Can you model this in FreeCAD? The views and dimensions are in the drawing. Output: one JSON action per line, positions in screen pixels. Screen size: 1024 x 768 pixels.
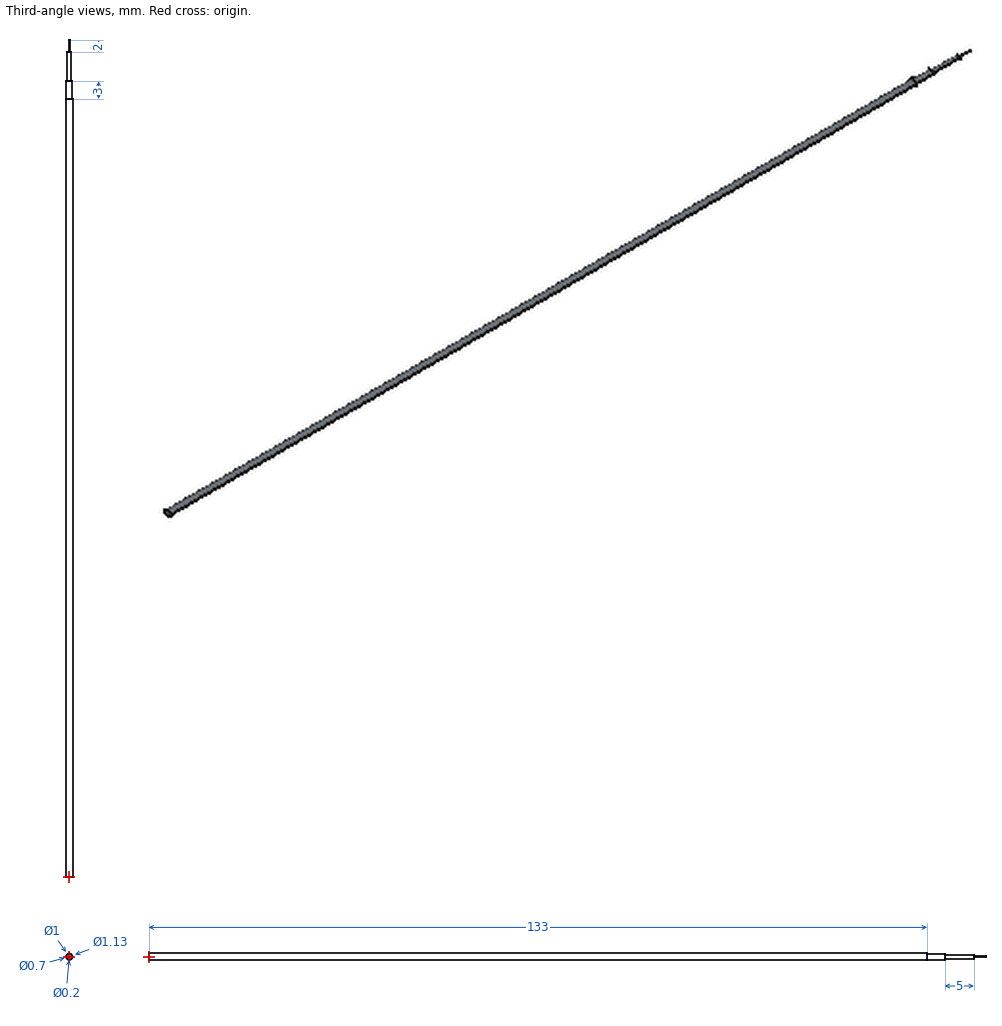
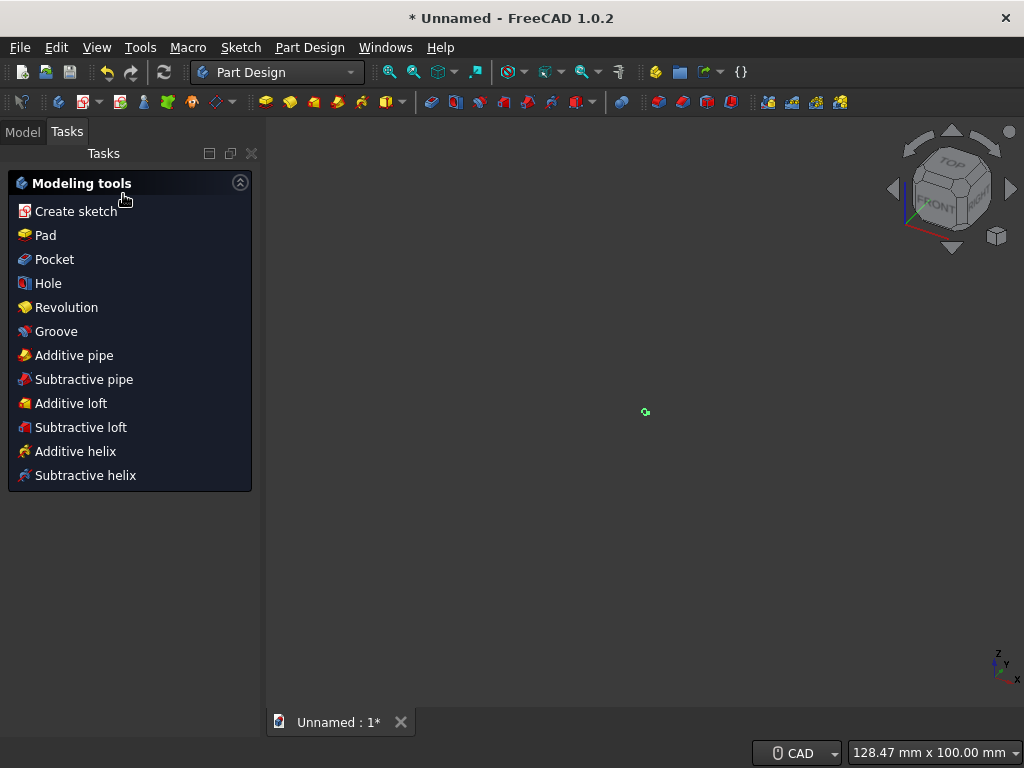
{"action": "left_click", "coordinate": [266, 102]}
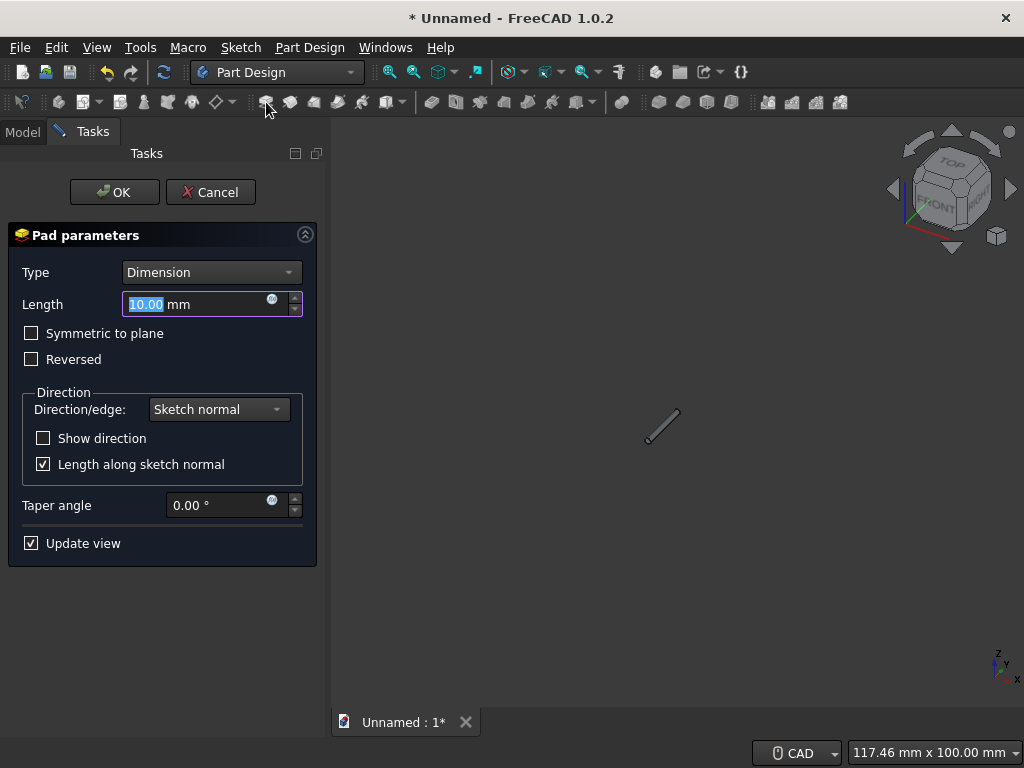
{"action": "type", "text": "133"}
{"action": "key", "text": "Tab"}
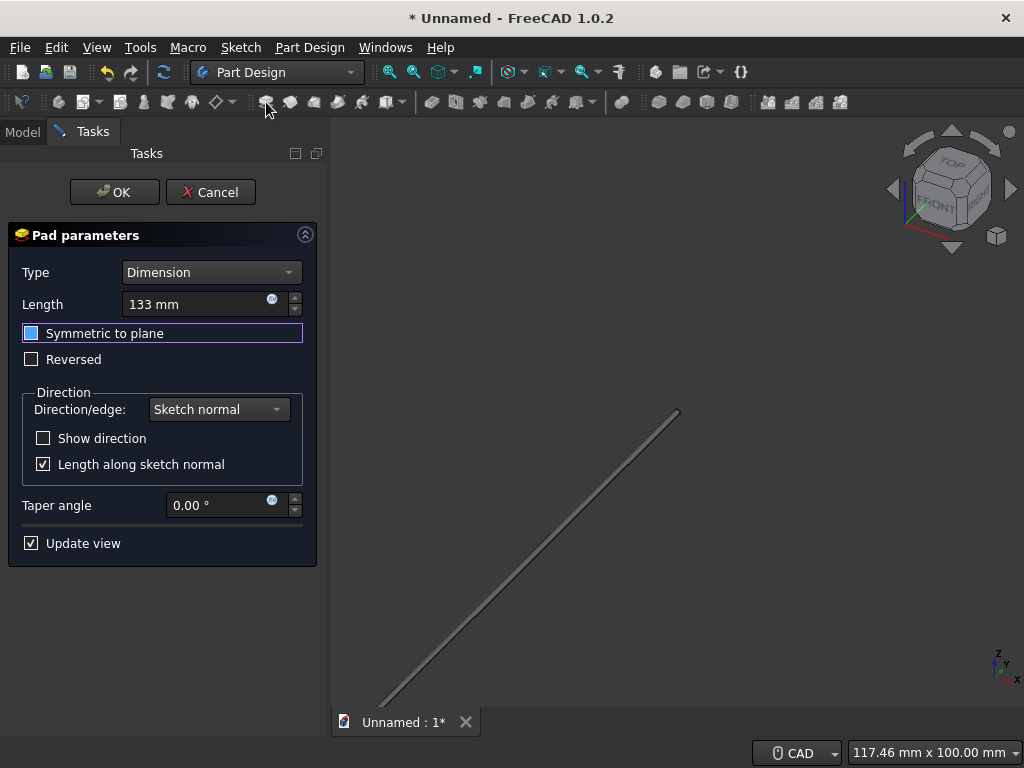
{"action": "left_click", "coordinate": [30, 359]}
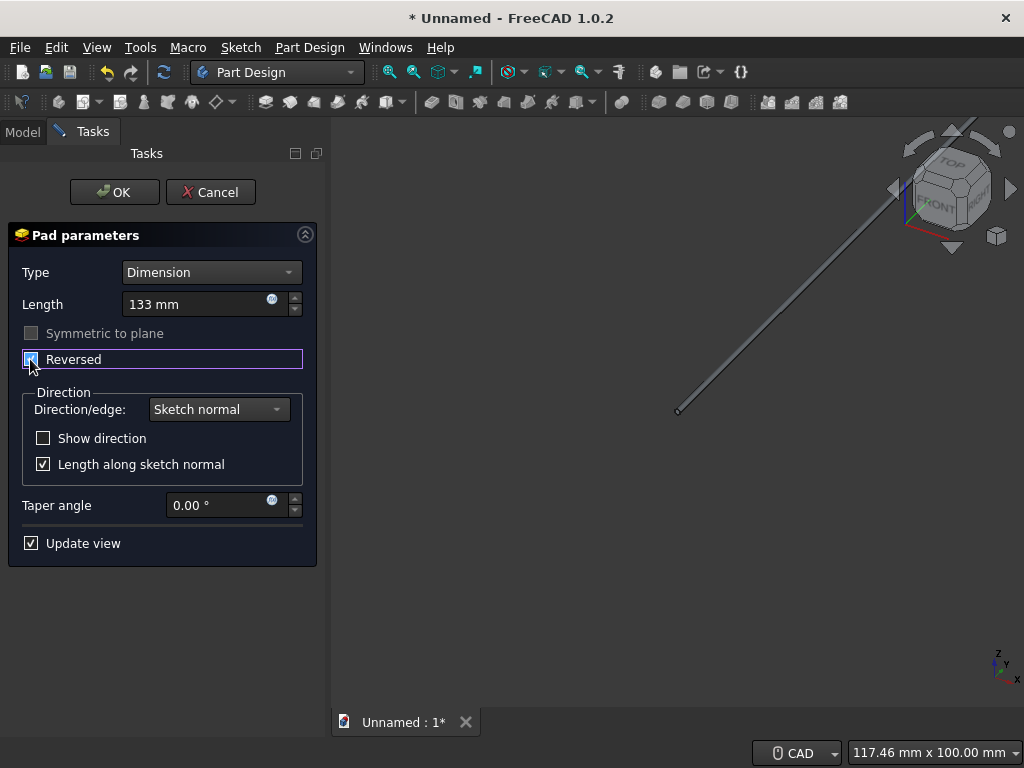
{"action": "left_click", "coordinate": [115, 192]}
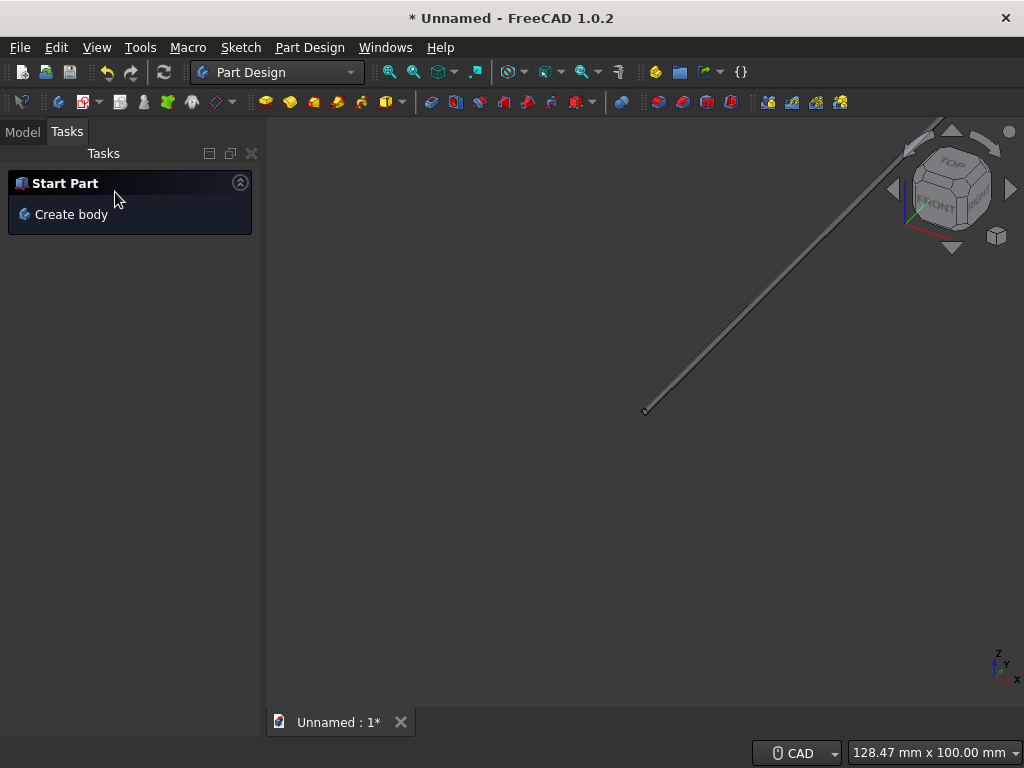
{"action": "left_click", "coordinate": [390, 72]}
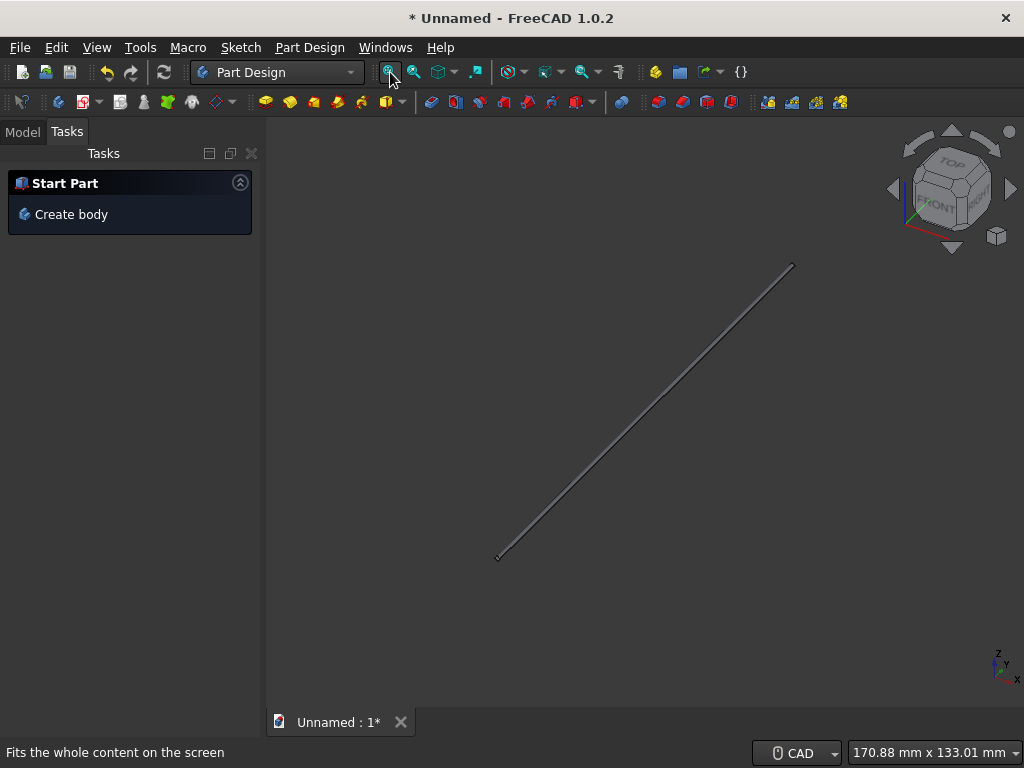
{"action": "key", "text": "4"}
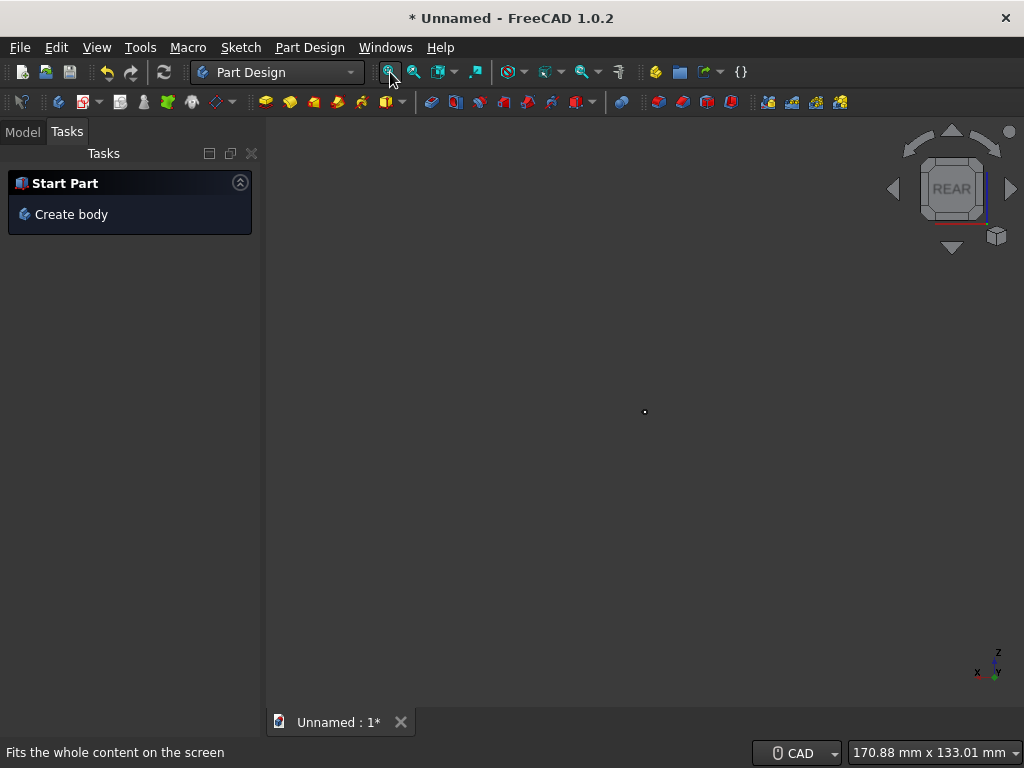
{"action": "left_click", "coordinate": [390, 72]}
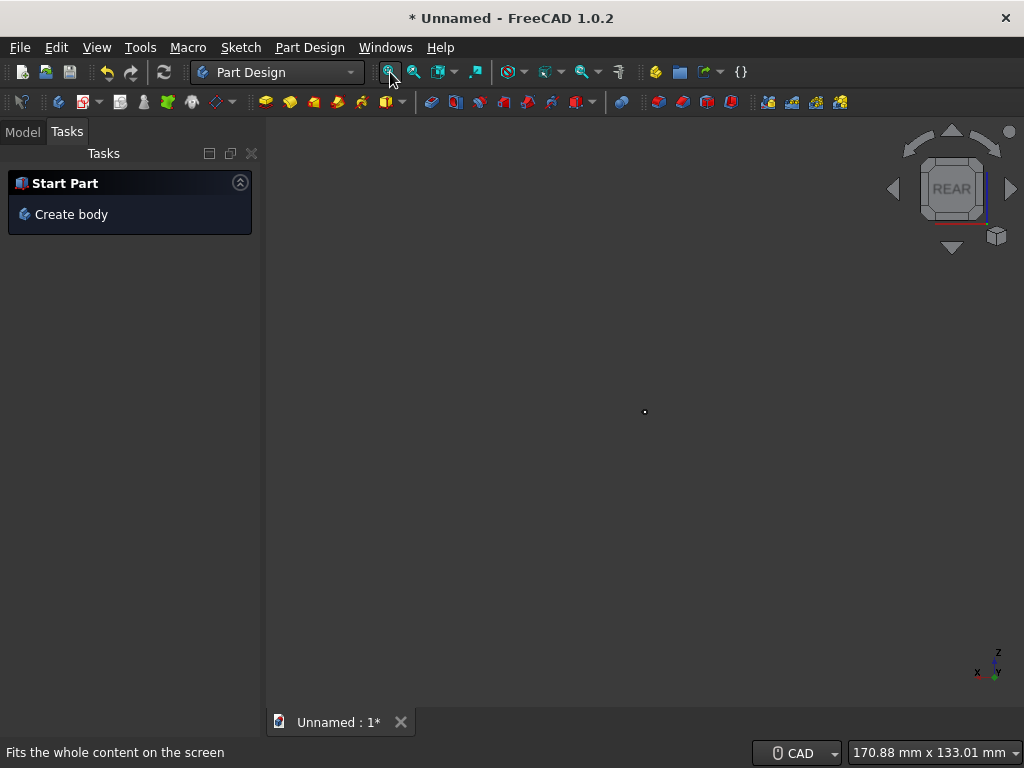
{"action": "scroll", "coordinate": [645, 411], "scroll_direction": "up", "scroll_amount": 8}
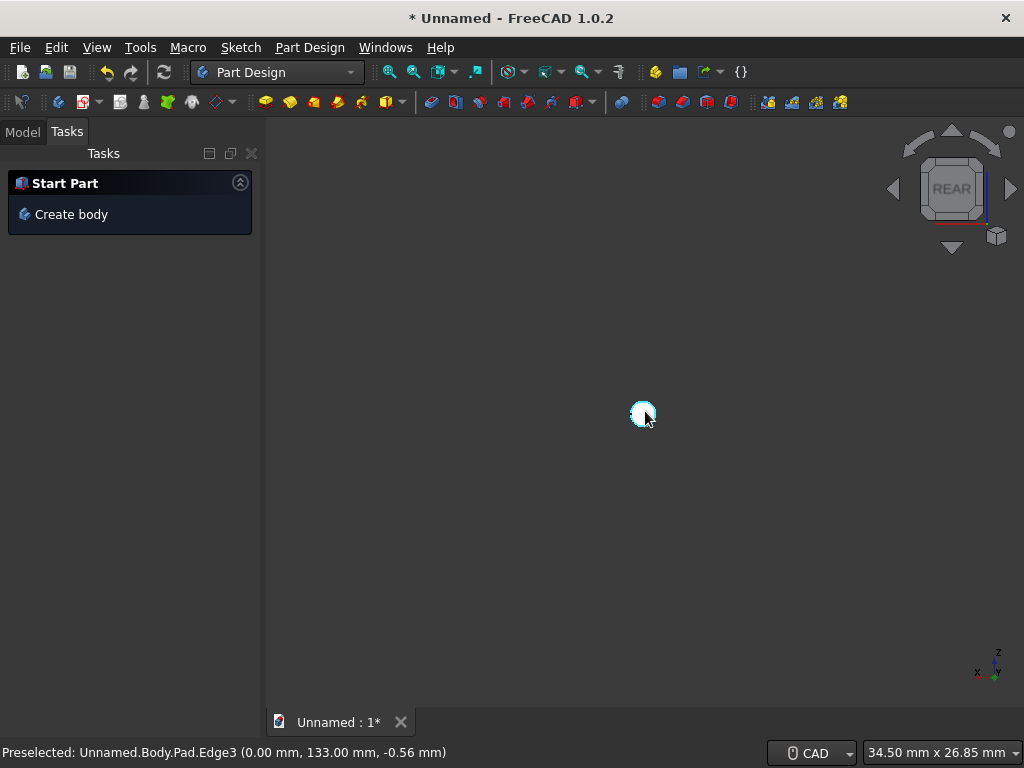
{"action": "left_click", "coordinate": [643, 413]}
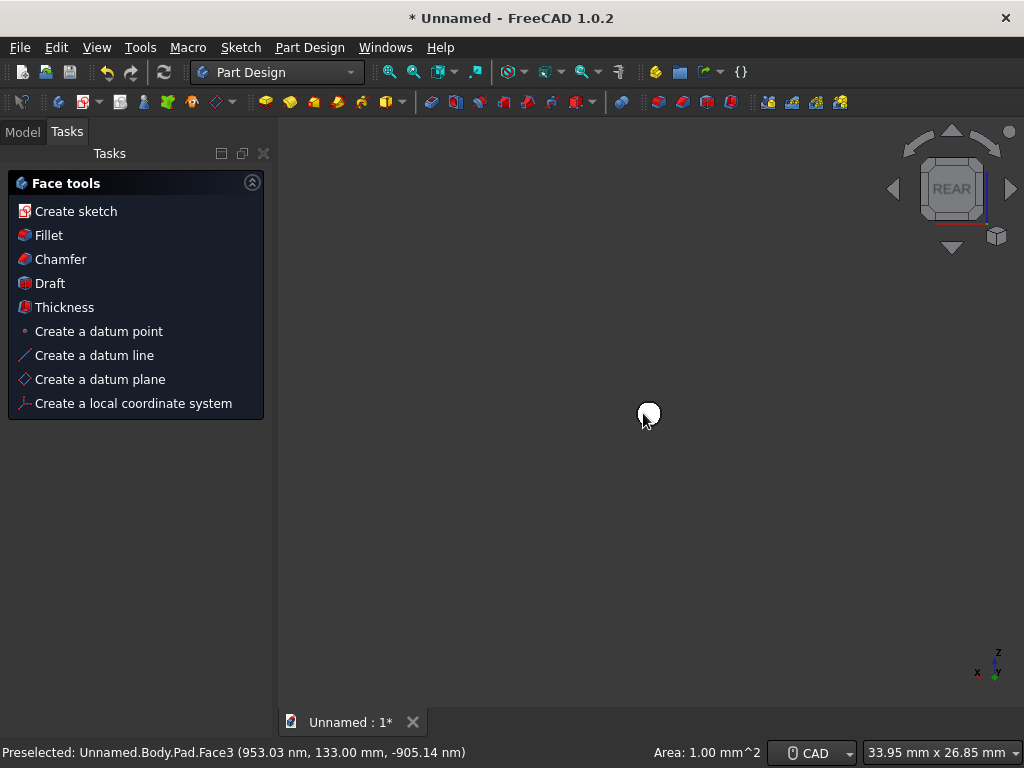
{"action": "left_click", "coordinate": [84, 102]}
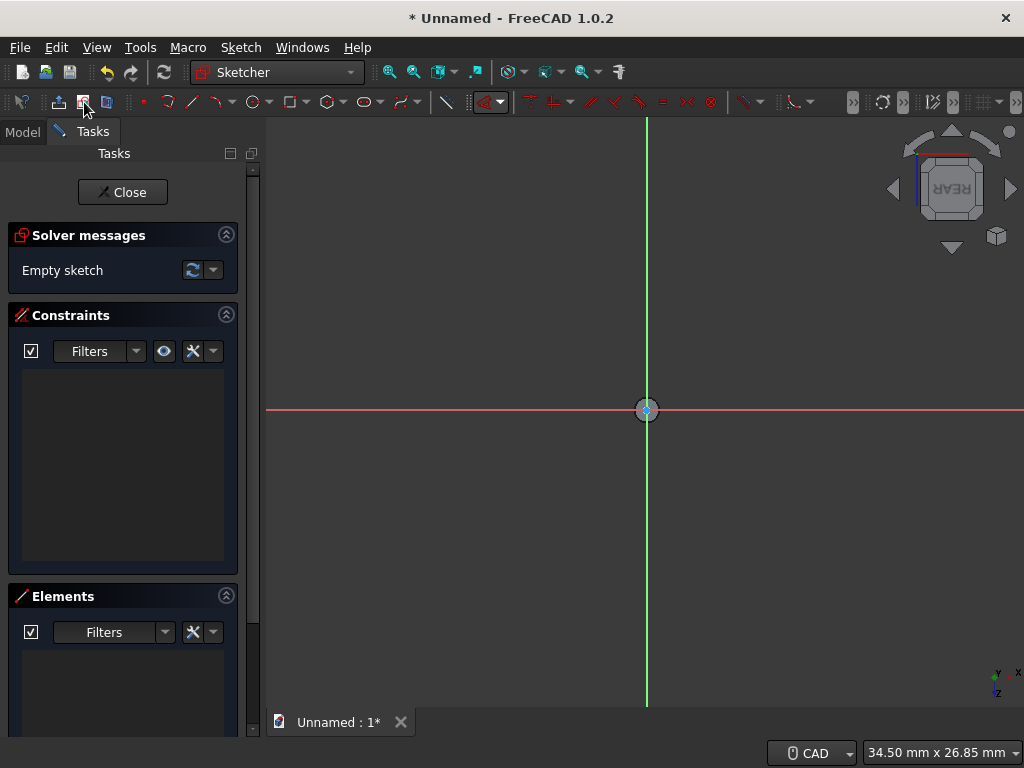
{"action": "scroll", "coordinate": [652, 410], "scroll_direction": "up", "scroll_amount": 14}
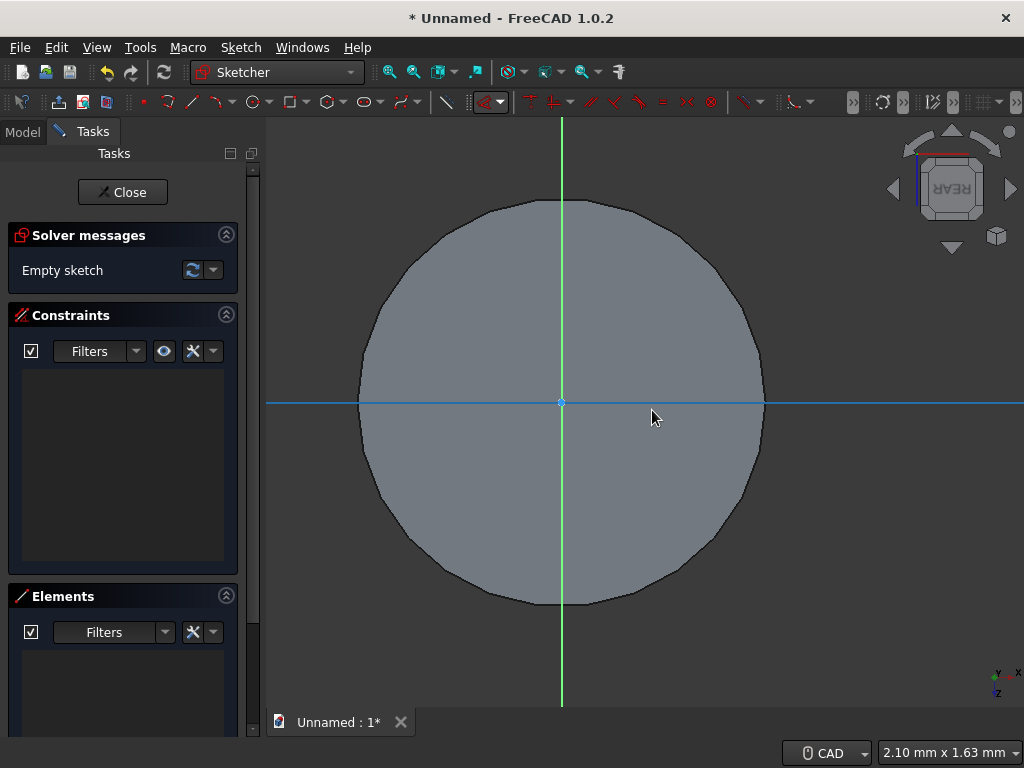
{"action": "key", "text": "g c"}